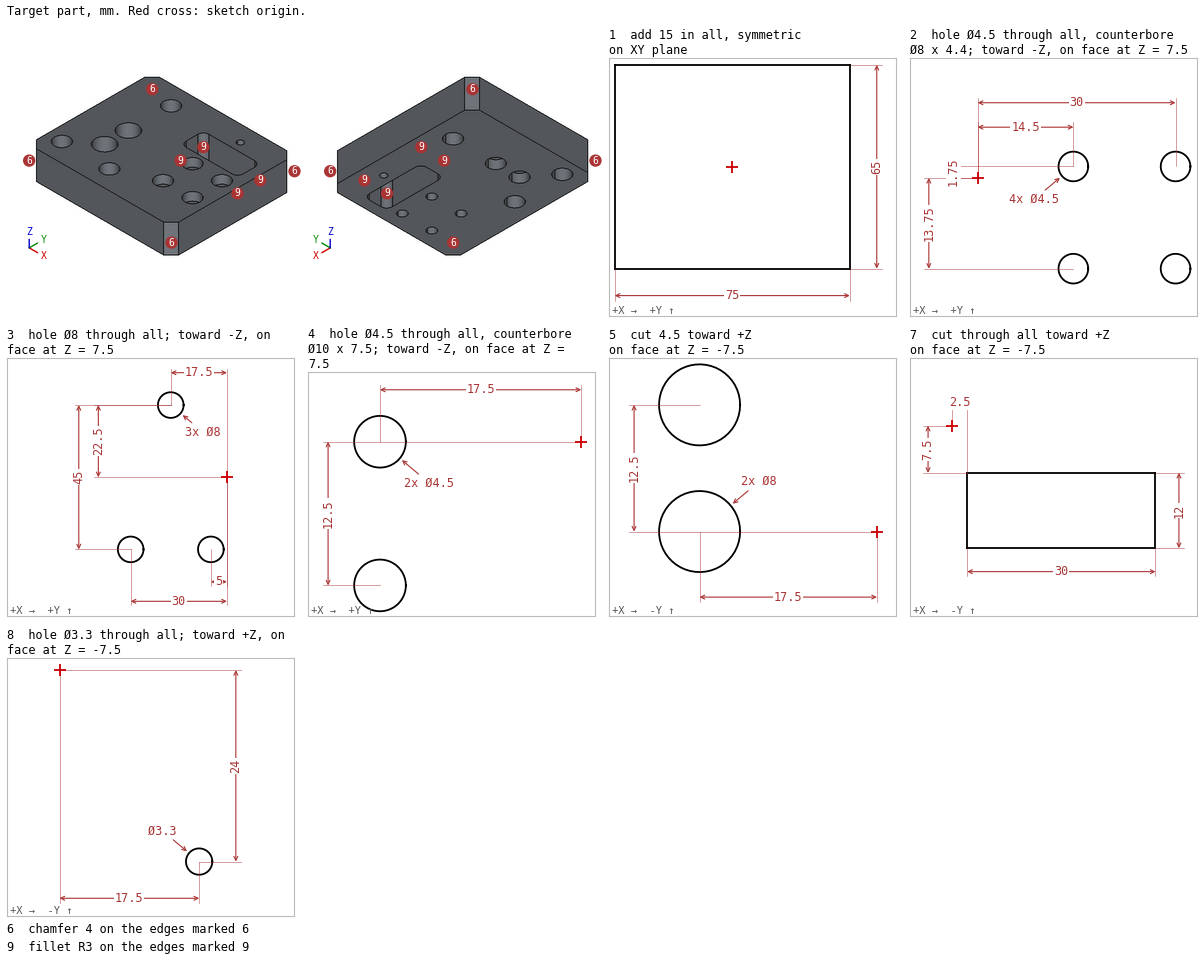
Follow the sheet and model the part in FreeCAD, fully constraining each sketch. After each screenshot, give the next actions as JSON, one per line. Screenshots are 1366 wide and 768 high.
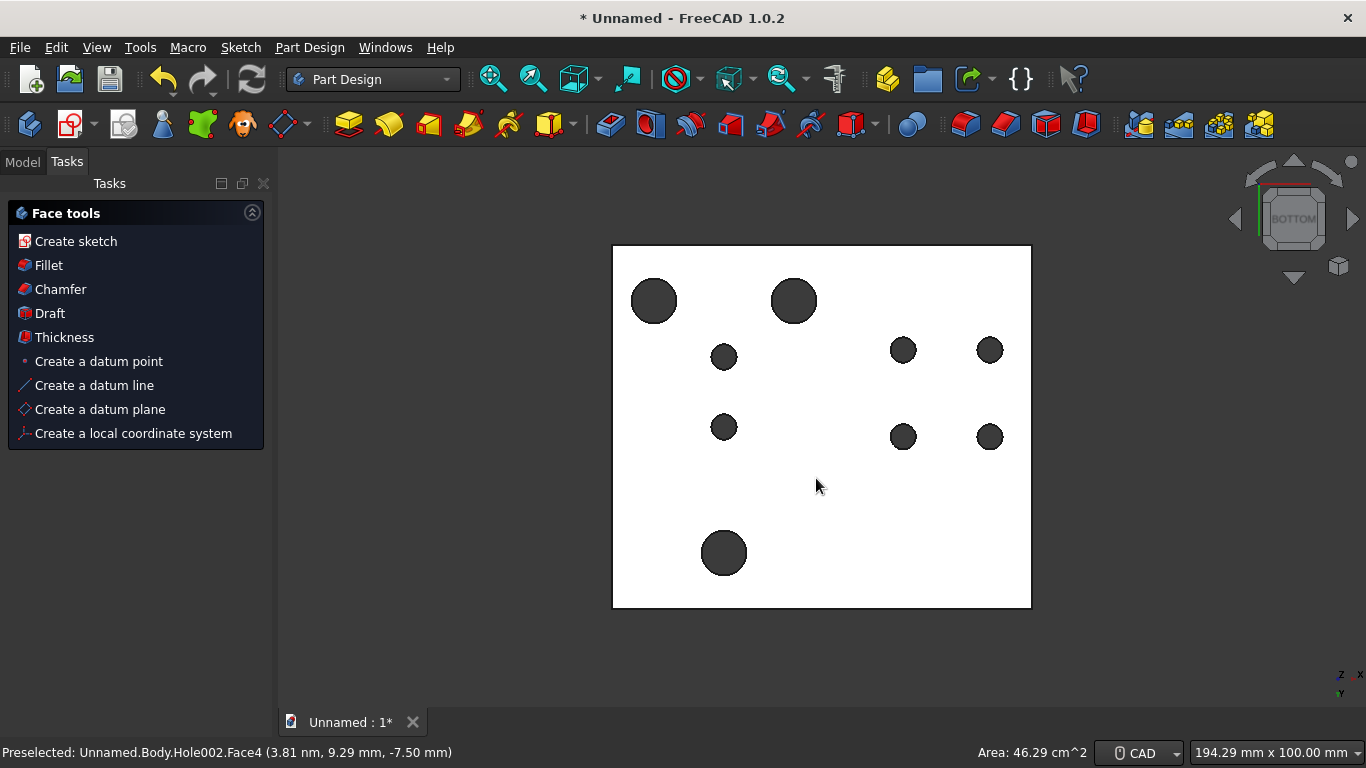
{"action": "left_click", "coordinate": [70, 124]}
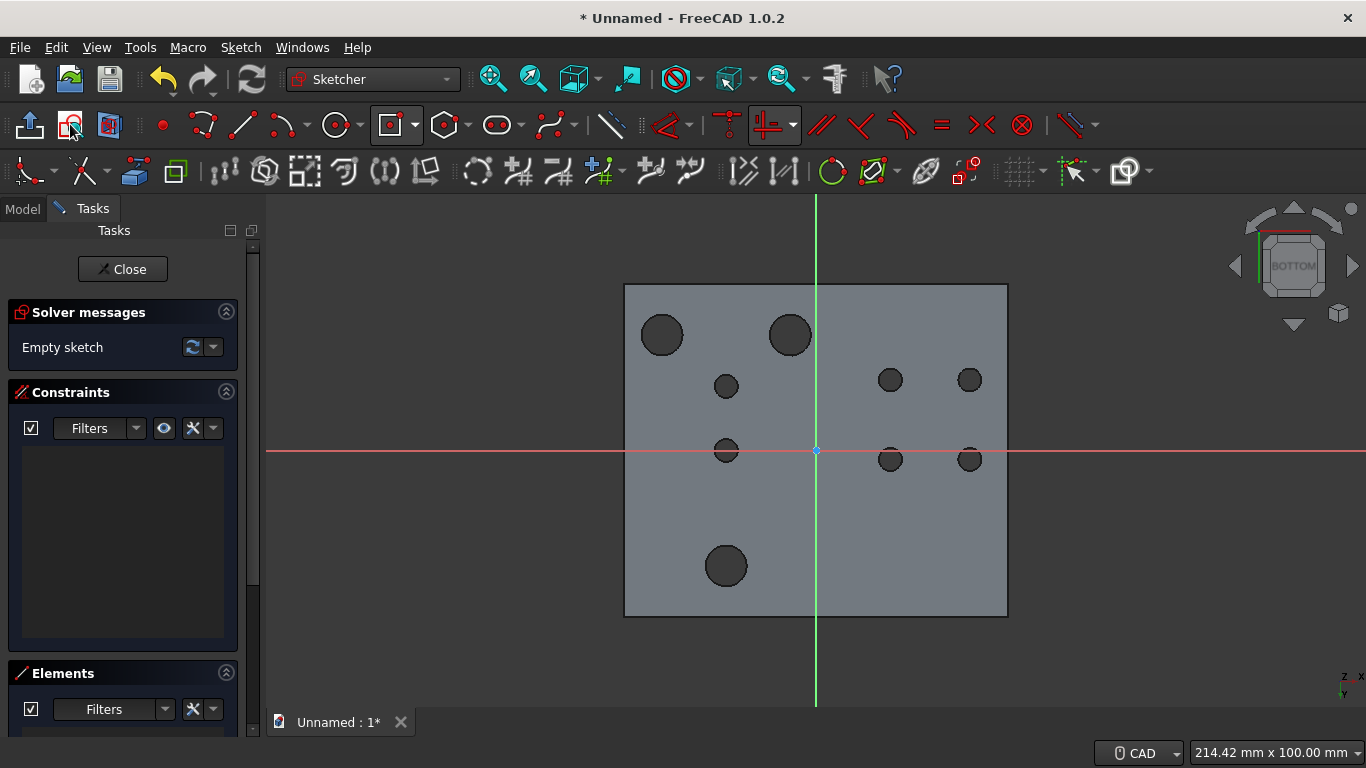
{"action": "scroll", "coordinate": [767, 405], "scroll_direction": "up", "scroll_amount": 6}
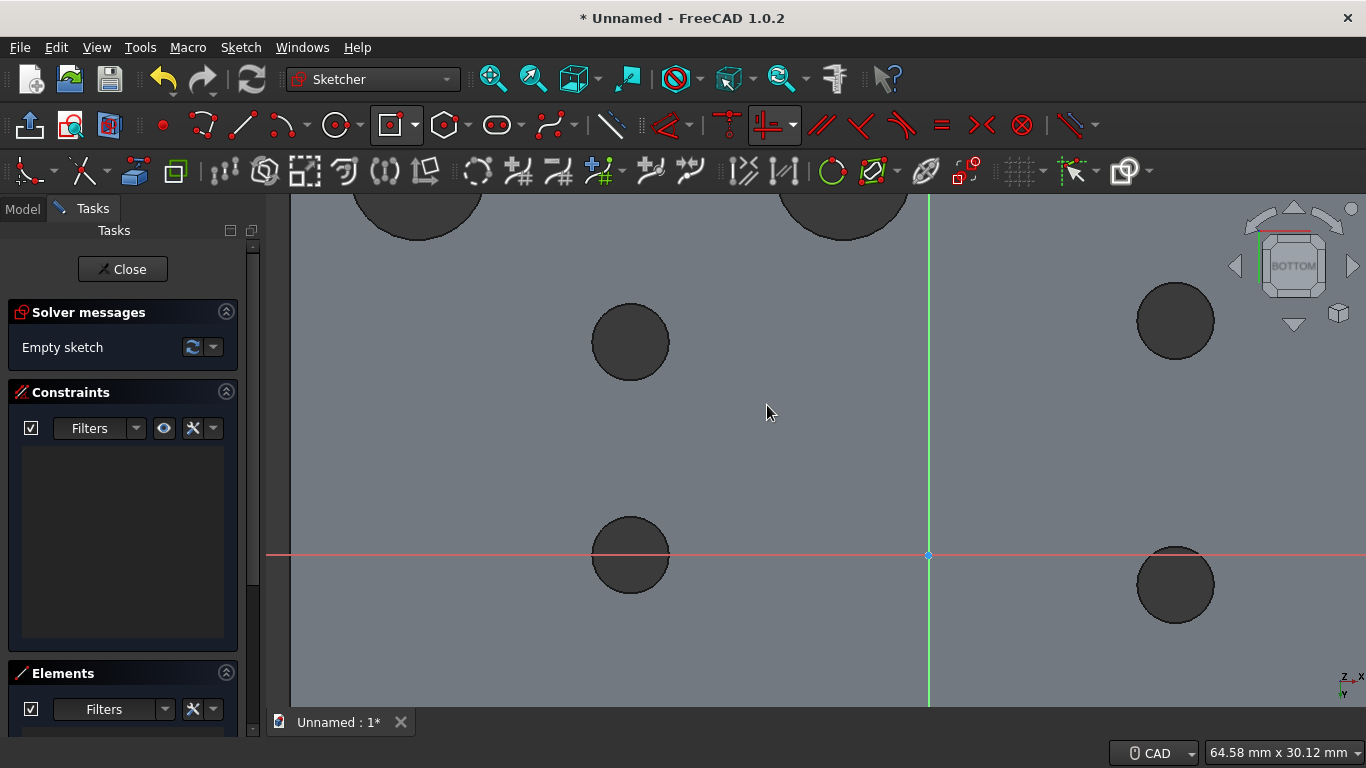
{"action": "key", "text": "g c"}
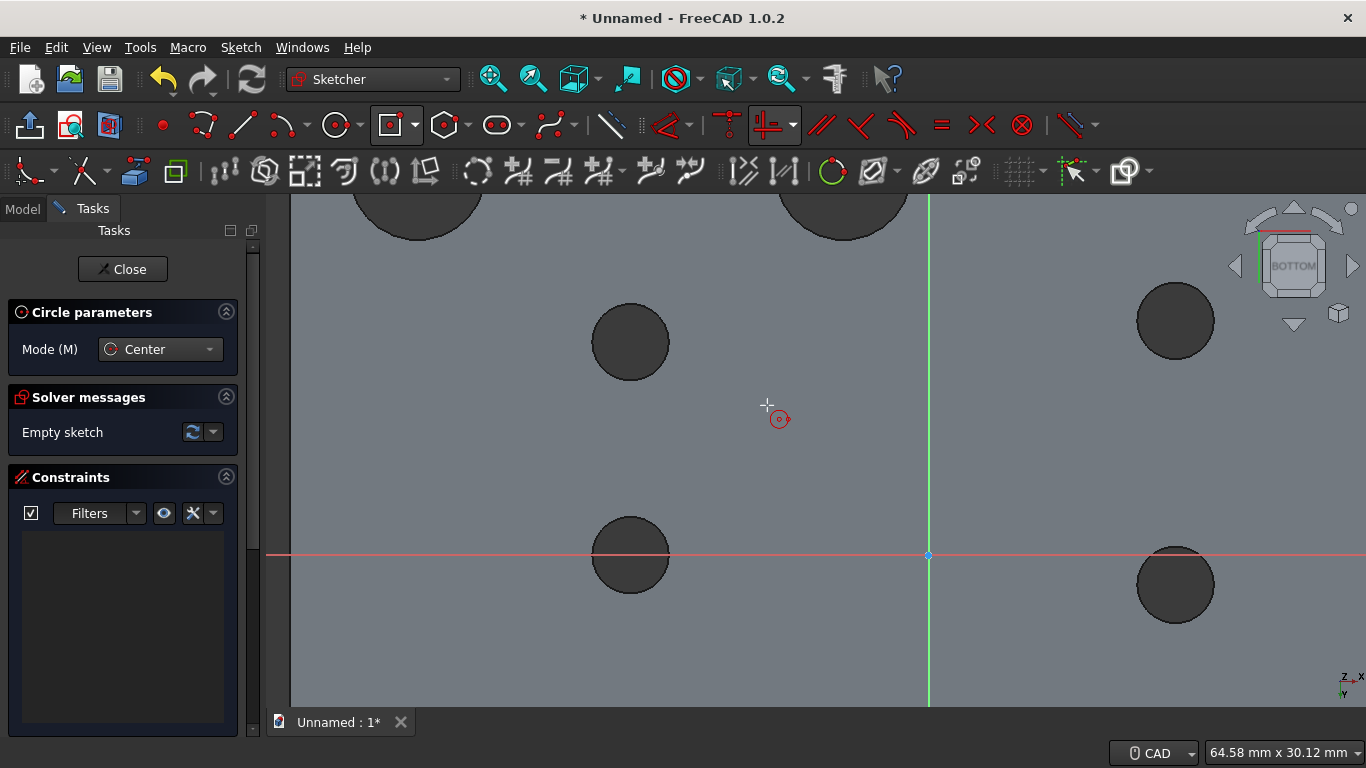
{"action": "left_click", "coordinate": [631, 555]}
{"action": "mouse_move", "coordinate": [679, 507]}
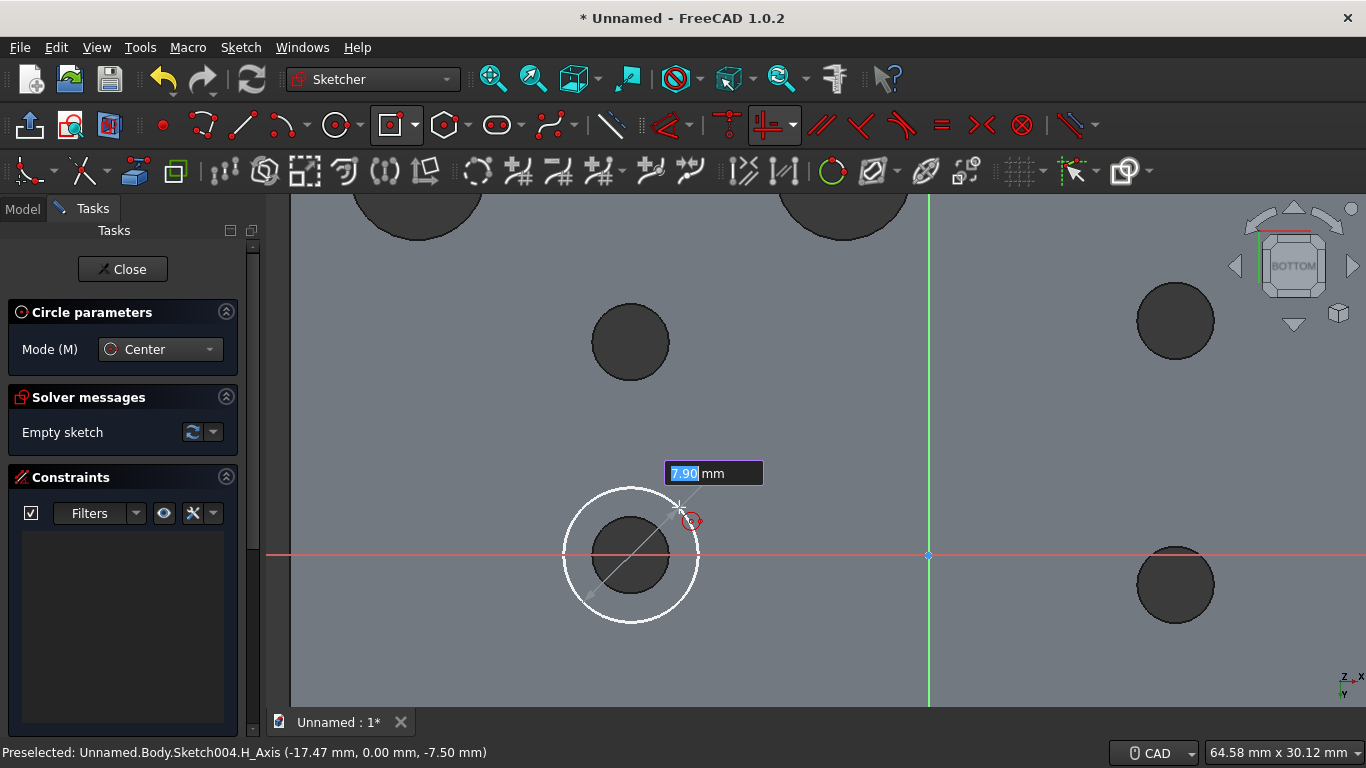
{"action": "type", "text": "8"}
{"action": "key", "text": "Return"}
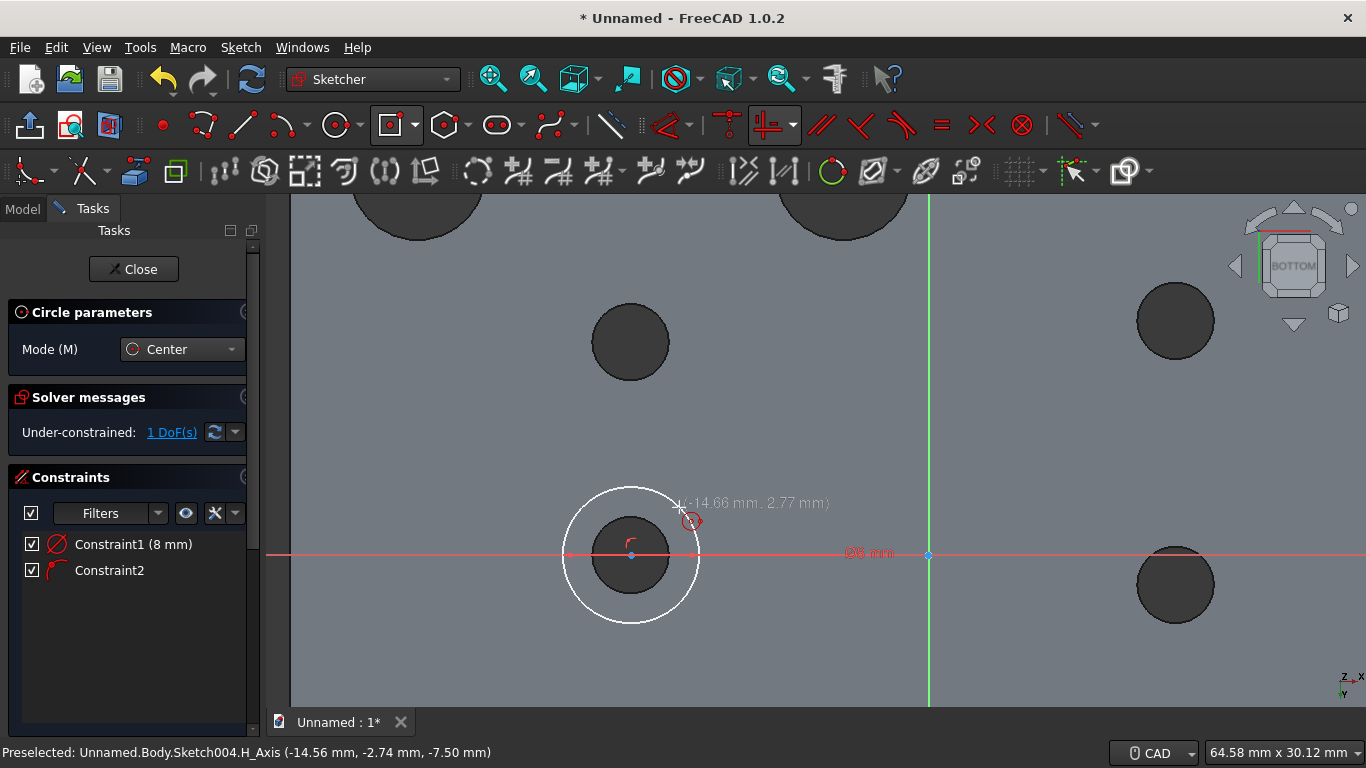
{"action": "left_click", "coordinate": [631, 342]}
{"action": "mouse_move", "coordinate": [679, 294]}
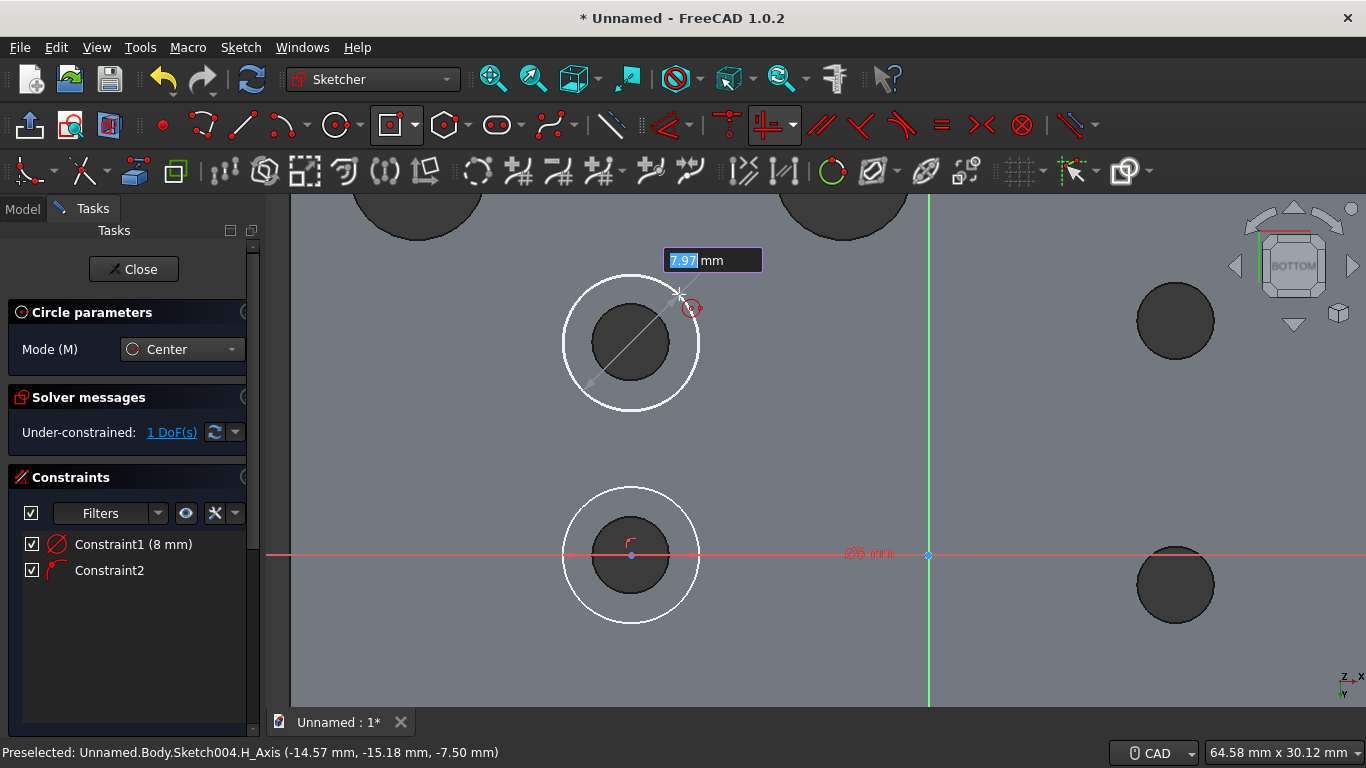
{"action": "type", "text": "8"}
{"action": "key", "text": "Return"}
{"action": "key", "text": "Escape"}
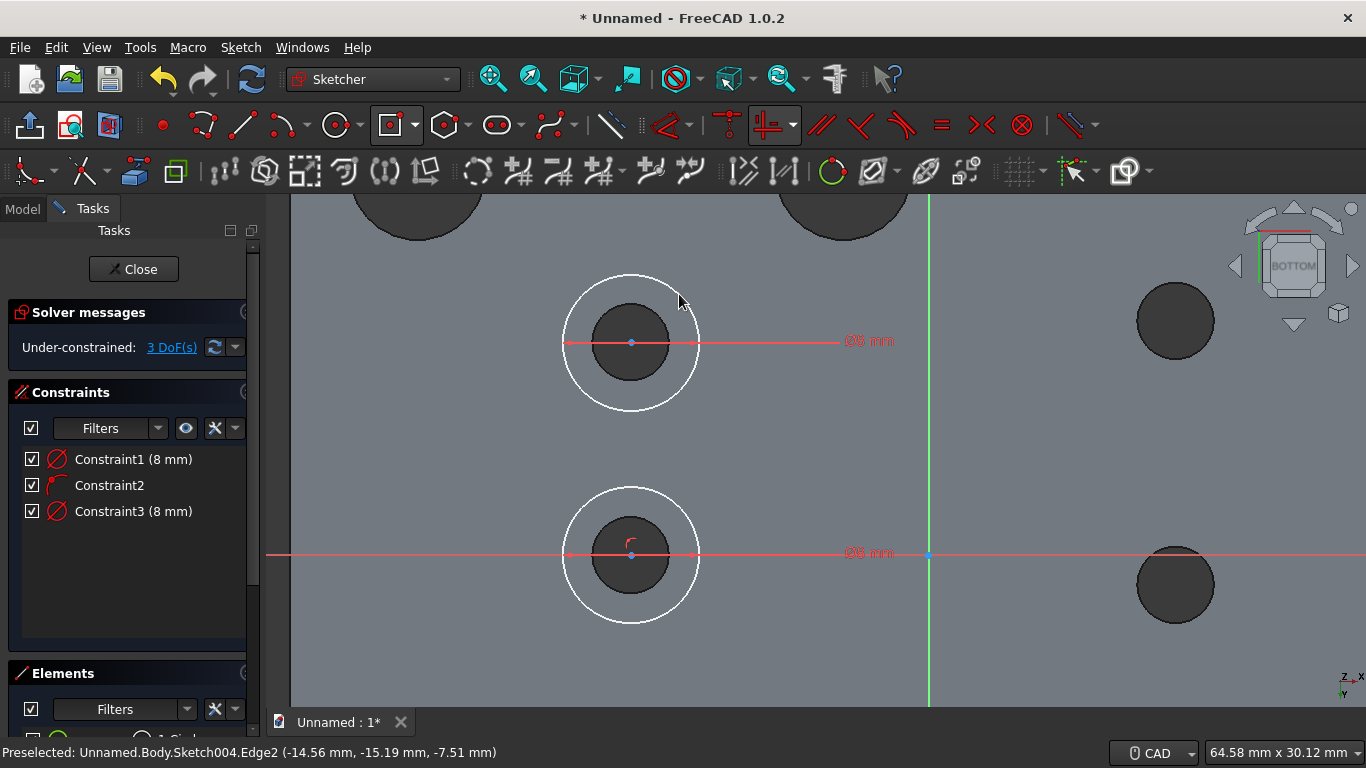
{"action": "left_click", "coordinate": [631, 555]}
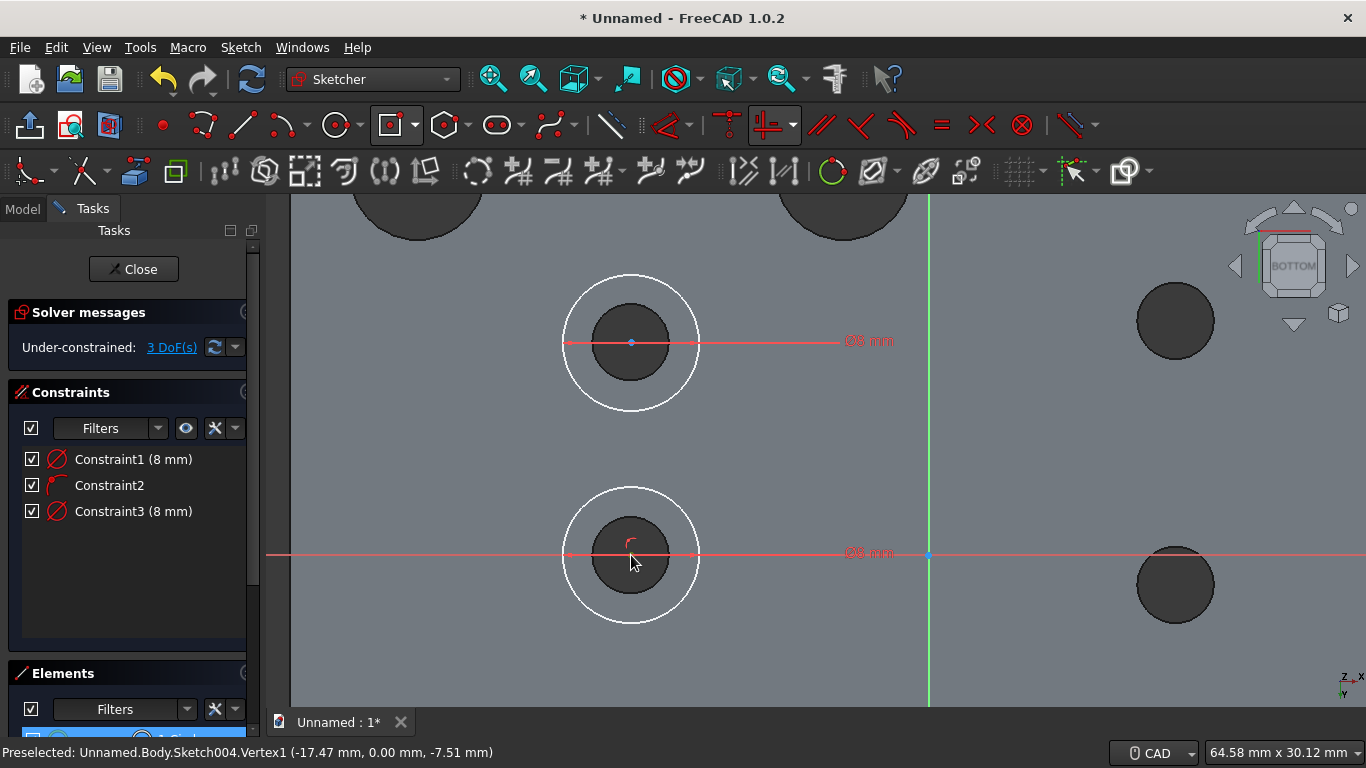
{"action": "left_click", "coordinate": [631, 343]}